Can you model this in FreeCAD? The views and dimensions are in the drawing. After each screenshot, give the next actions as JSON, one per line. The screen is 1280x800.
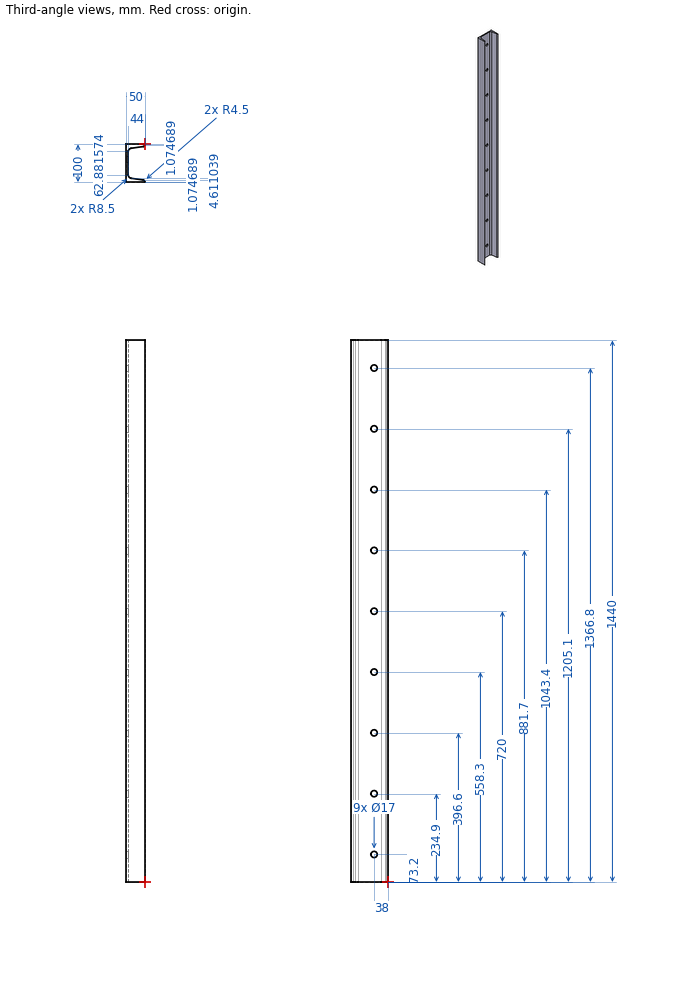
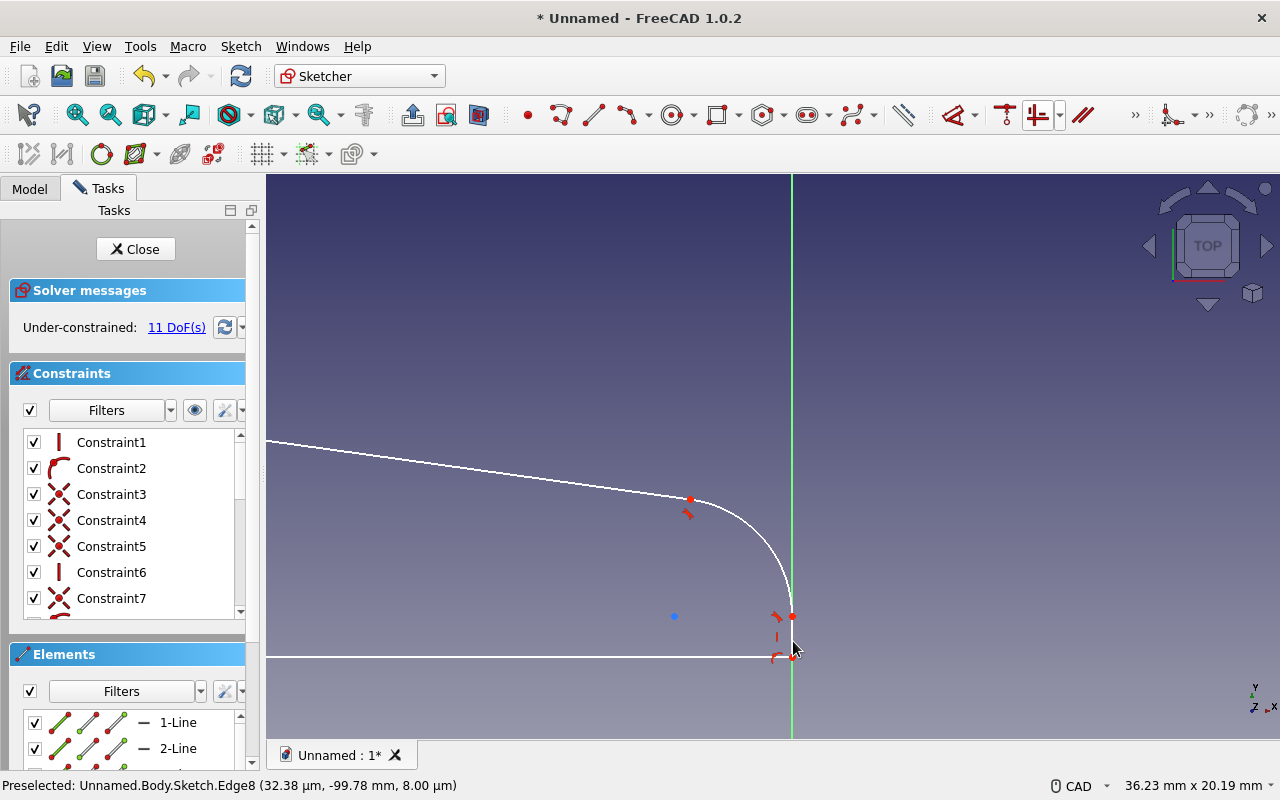
{"action": "scroll", "coordinate": [800, 645], "scroll_direction": "down", "scroll_amount": 10}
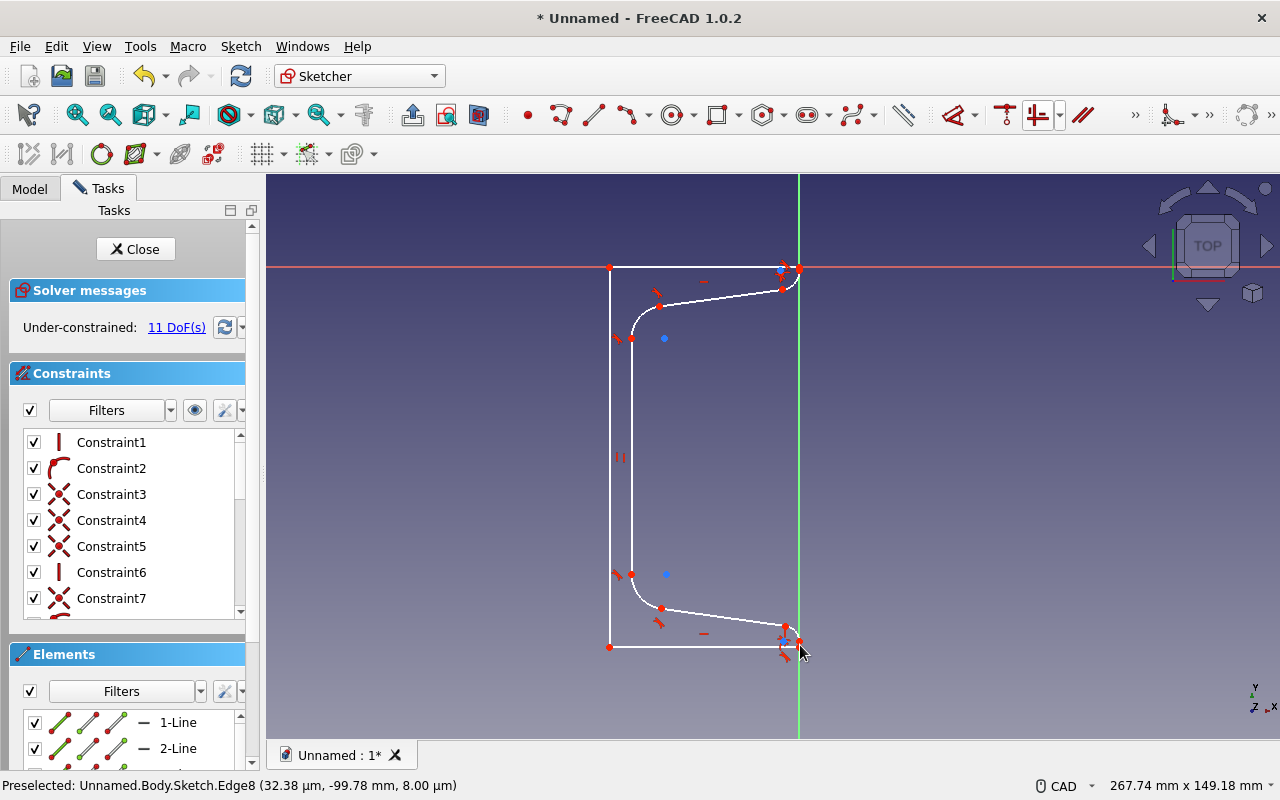
{"action": "left_click", "coordinate": [635, 589]}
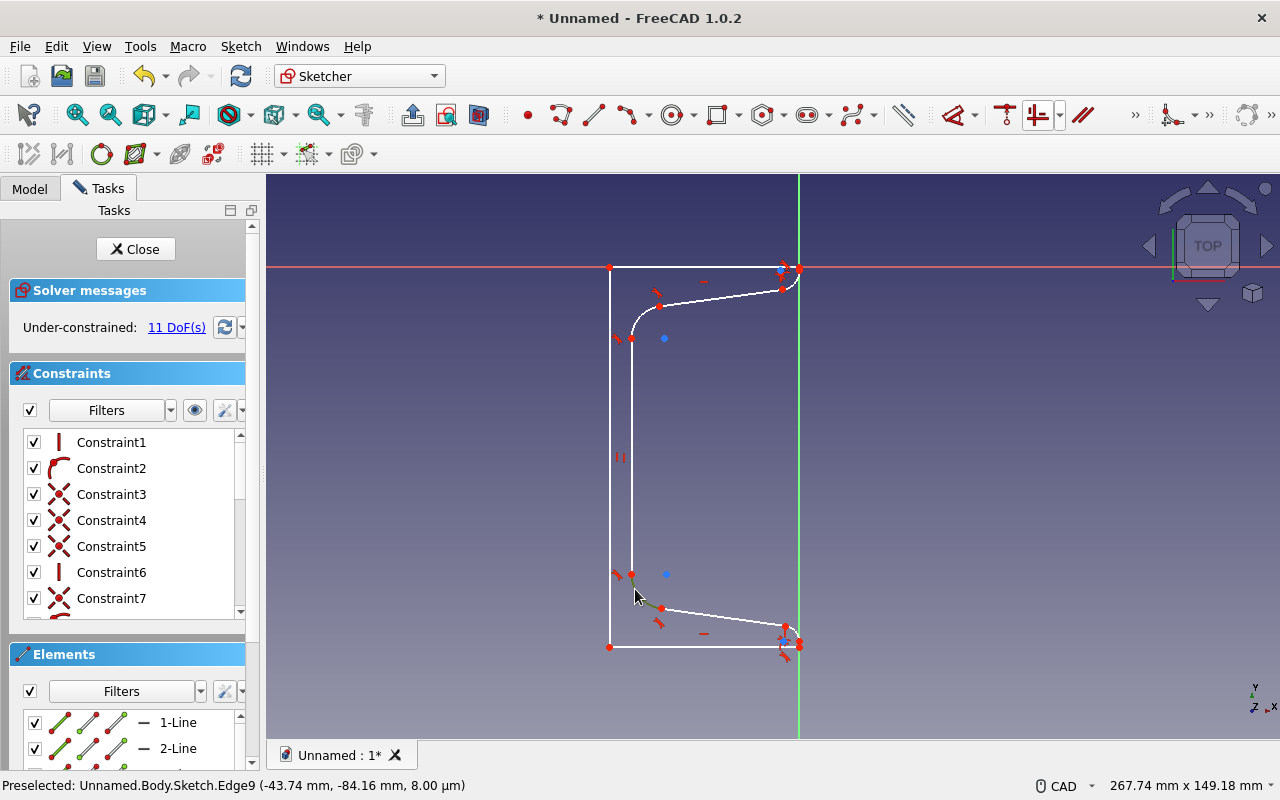
{"action": "left_click", "coordinate": [647, 311]}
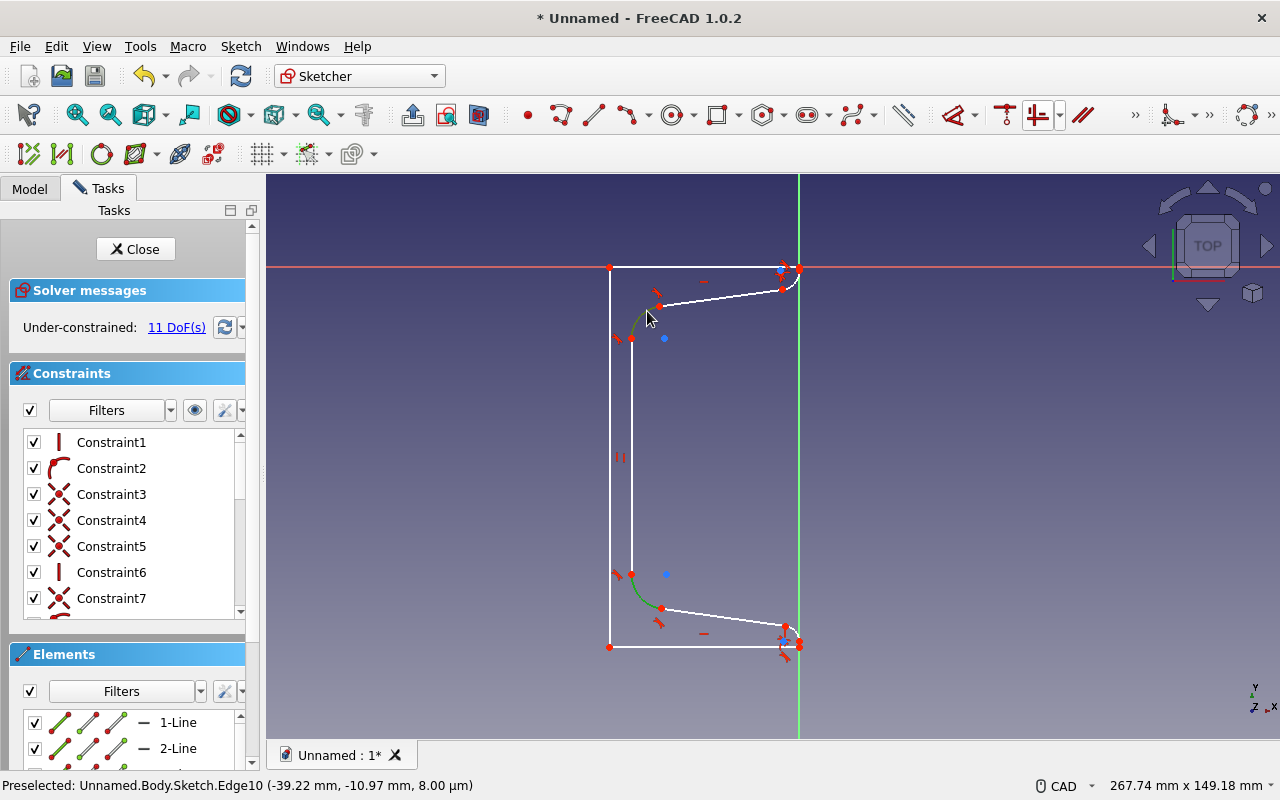
{"action": "key", "text": "e"}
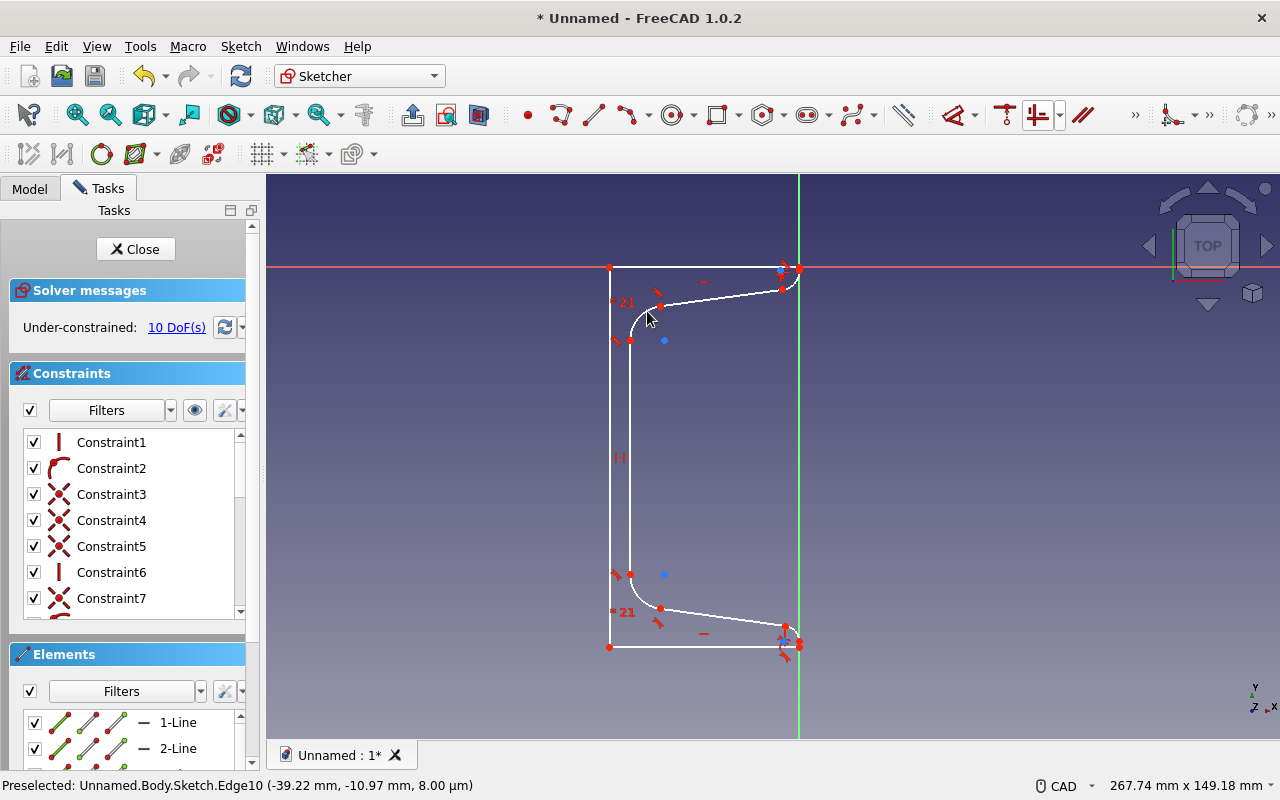
{"action": "scroll", "coordinate": [798, 279], "scroll_direction": "up", "scroll_amount": 3}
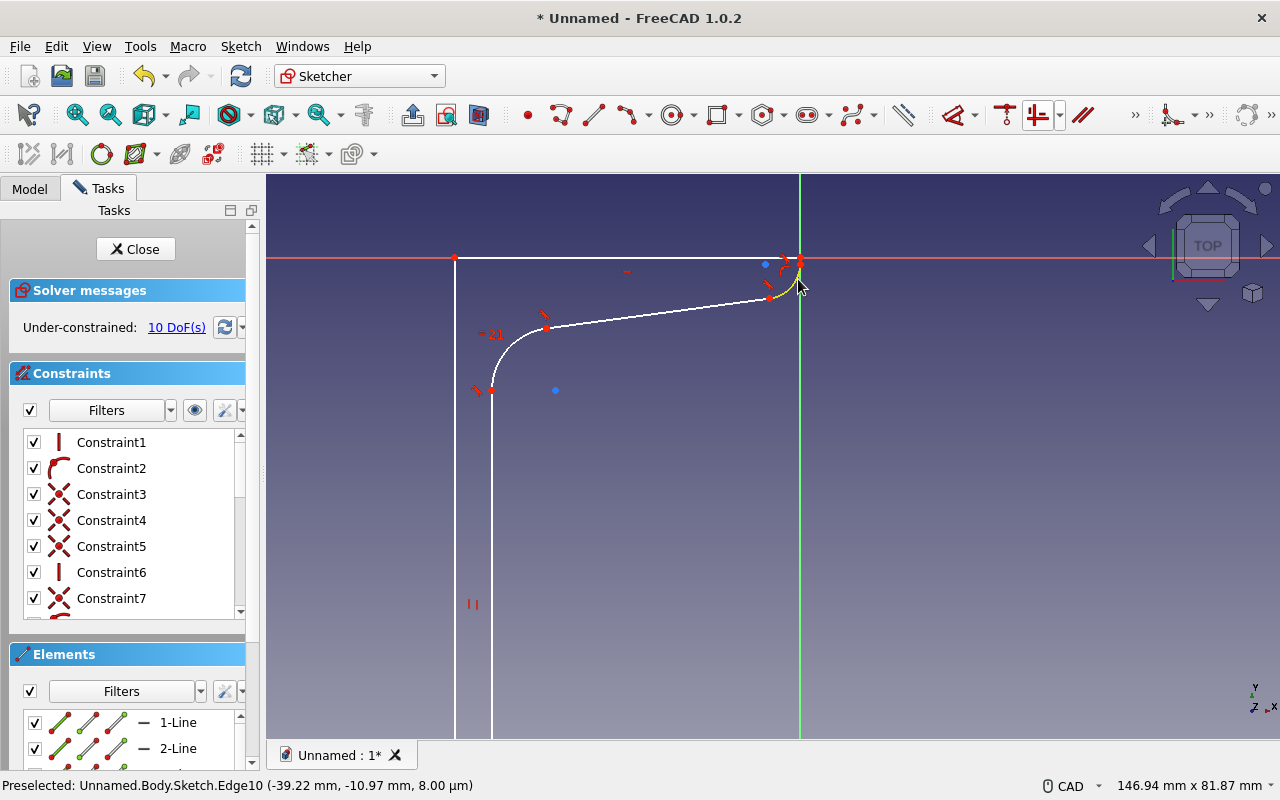
{"action": "left_click", "coordinate": [797, 279]}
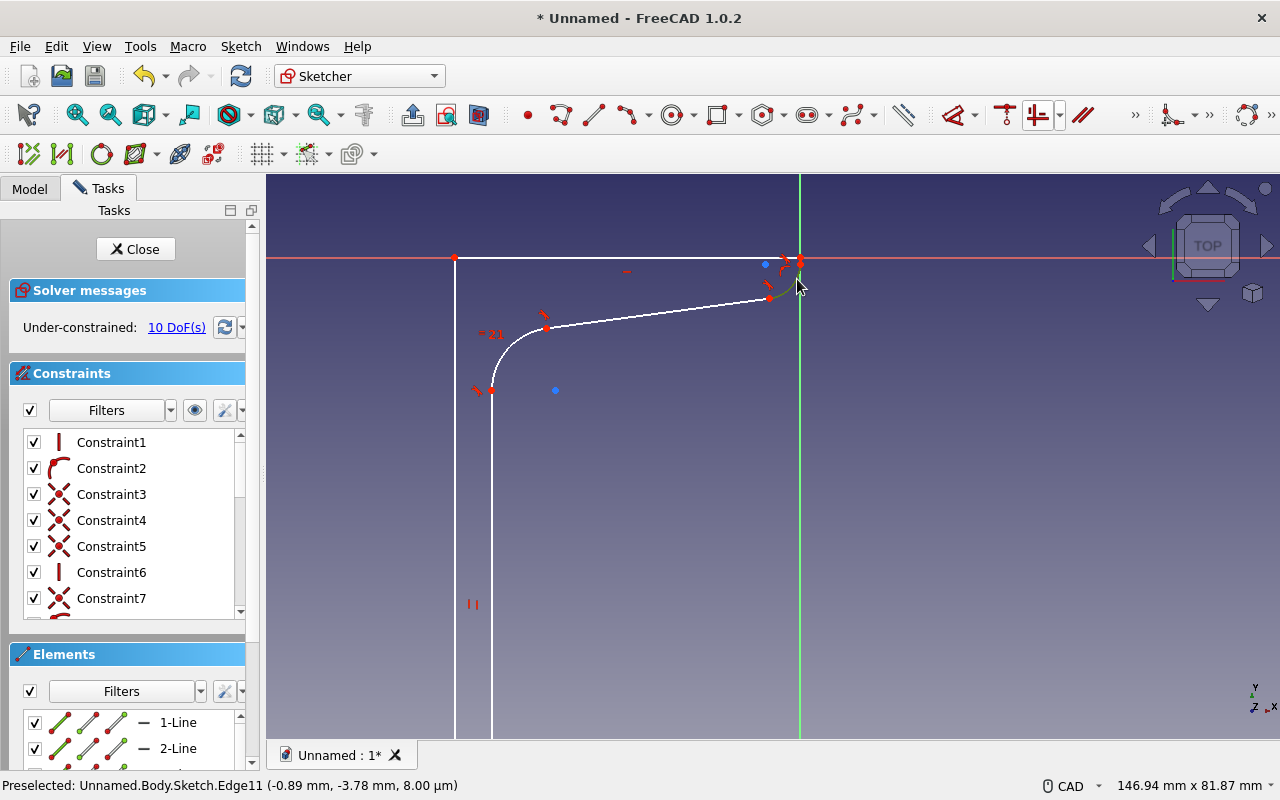
{"action": "scroll", "coordinate": [798, 279], "scroll_direction": "down", "scroll_amount": 3}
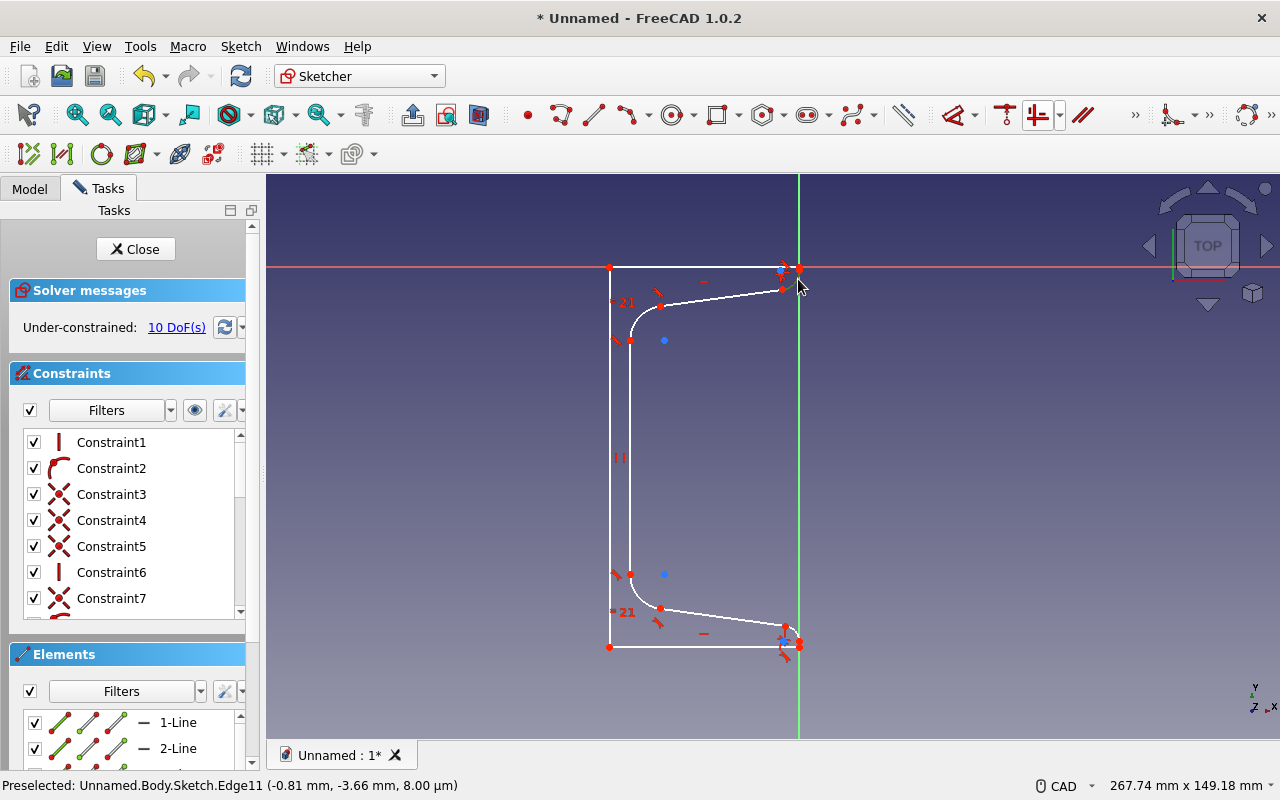
{"action": "scroll", "coordinate": [798, 635], "scroll_direction": "up", "scroll_amount": 4}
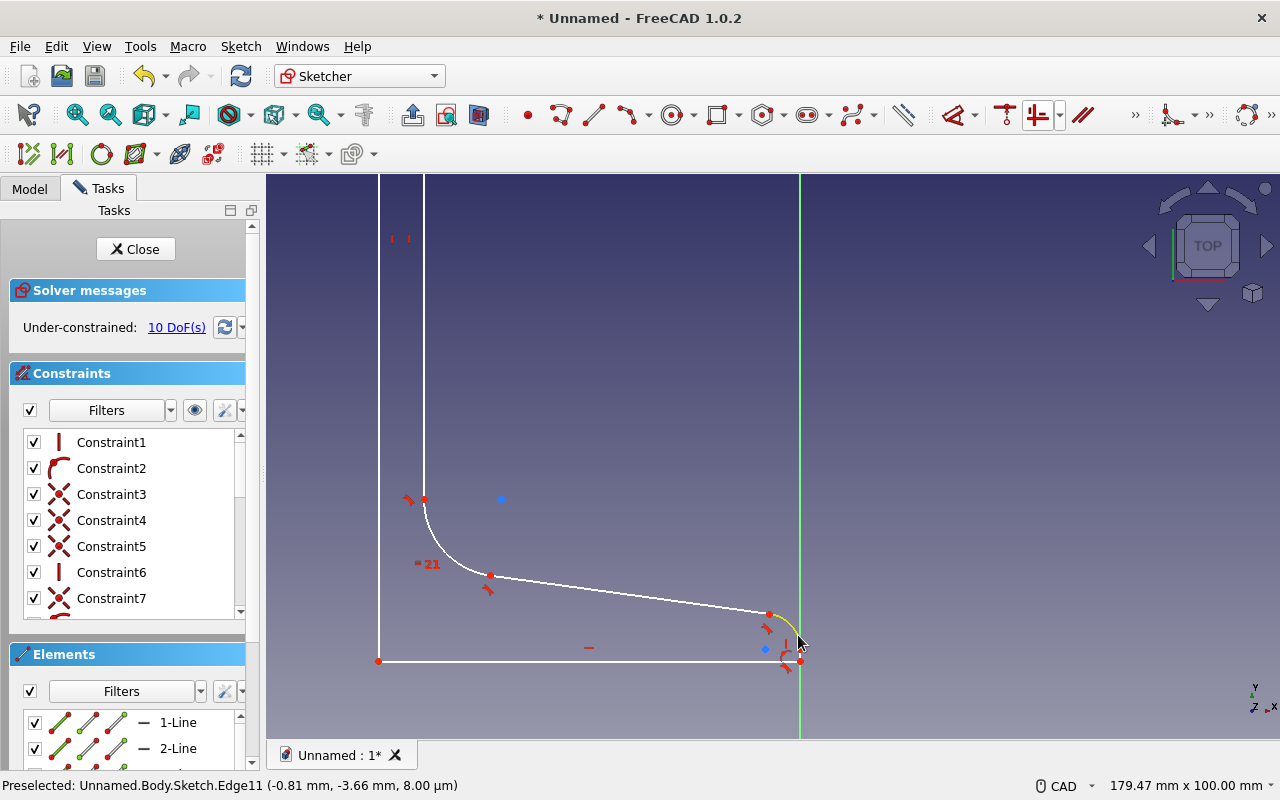
{"action": "left_click", "coordinate": [797, 634]}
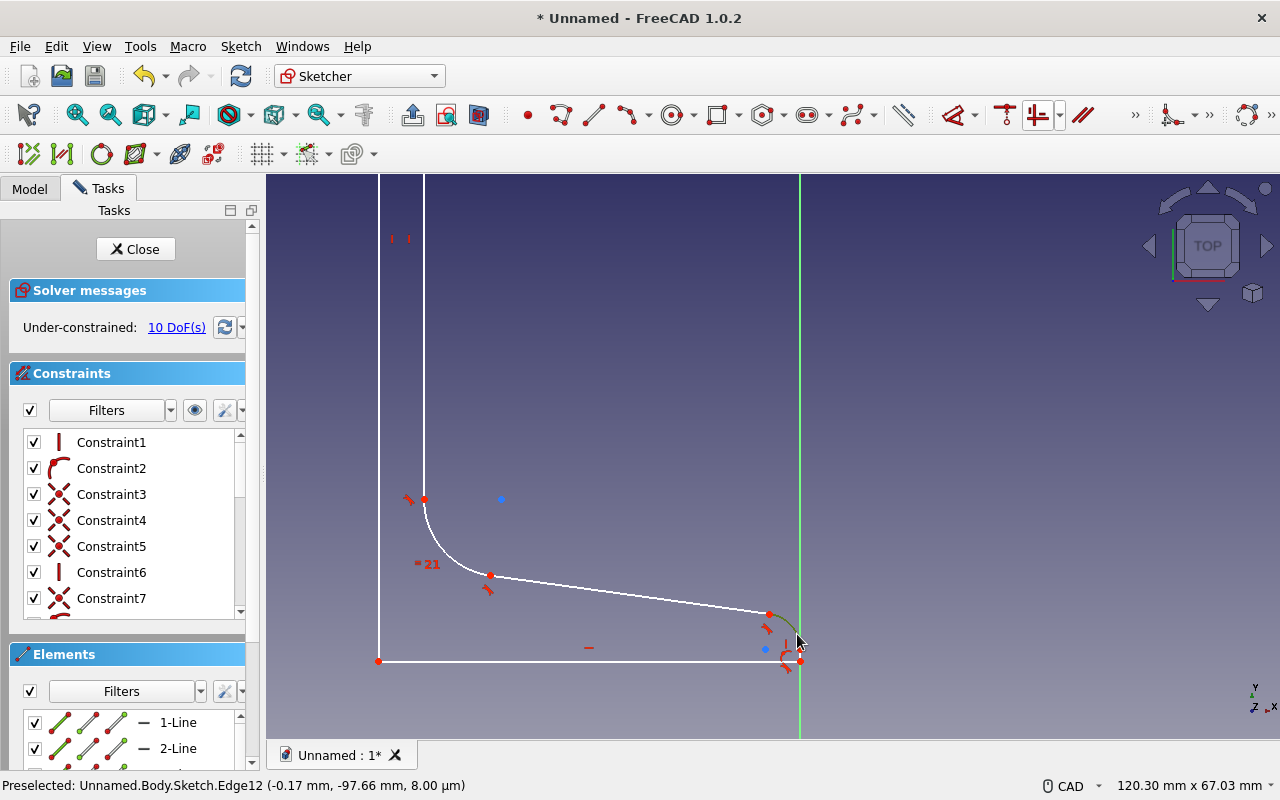
{"action": "key", "text": "e"}